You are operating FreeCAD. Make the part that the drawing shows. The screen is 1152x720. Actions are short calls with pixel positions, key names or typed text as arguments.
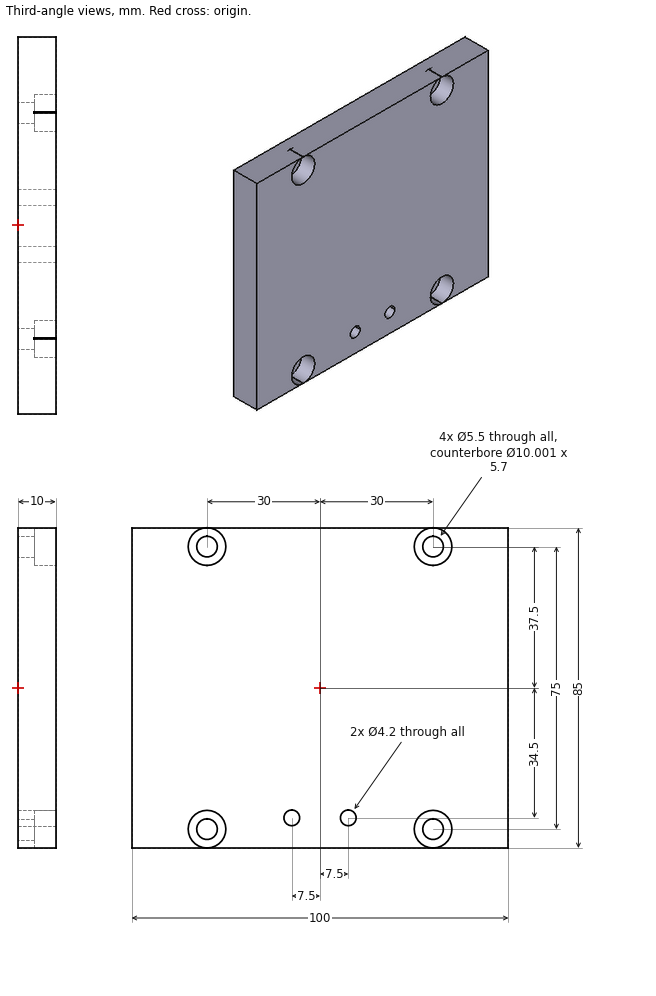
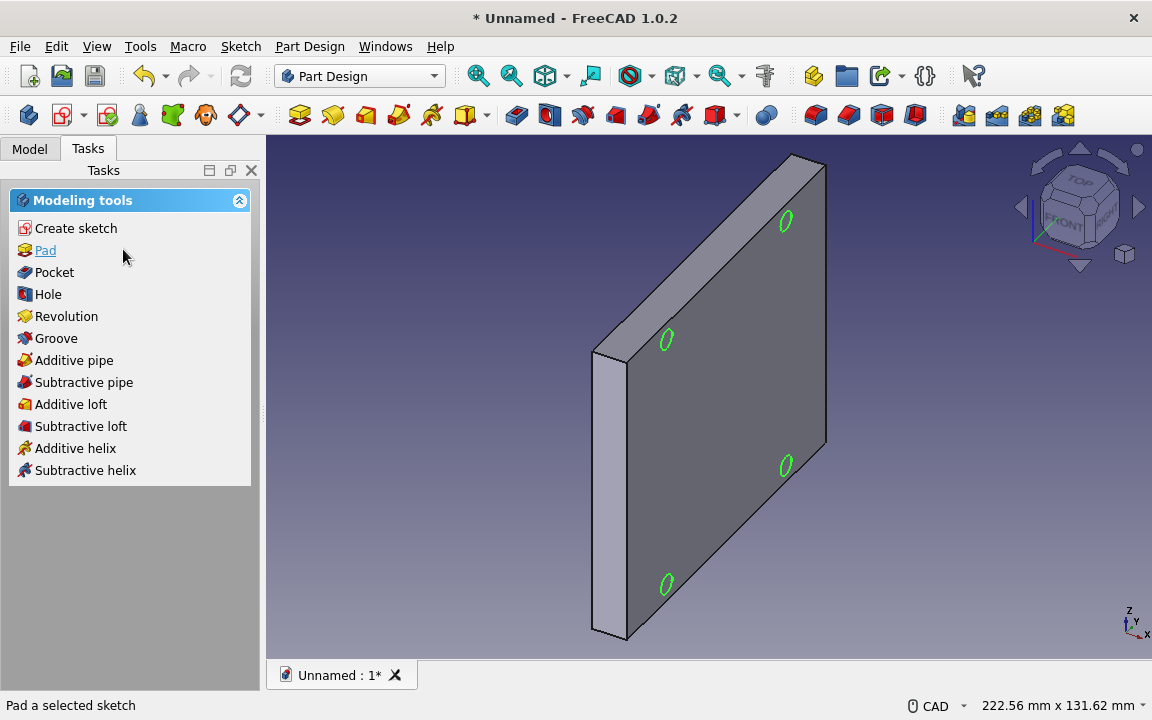
click(550, 116)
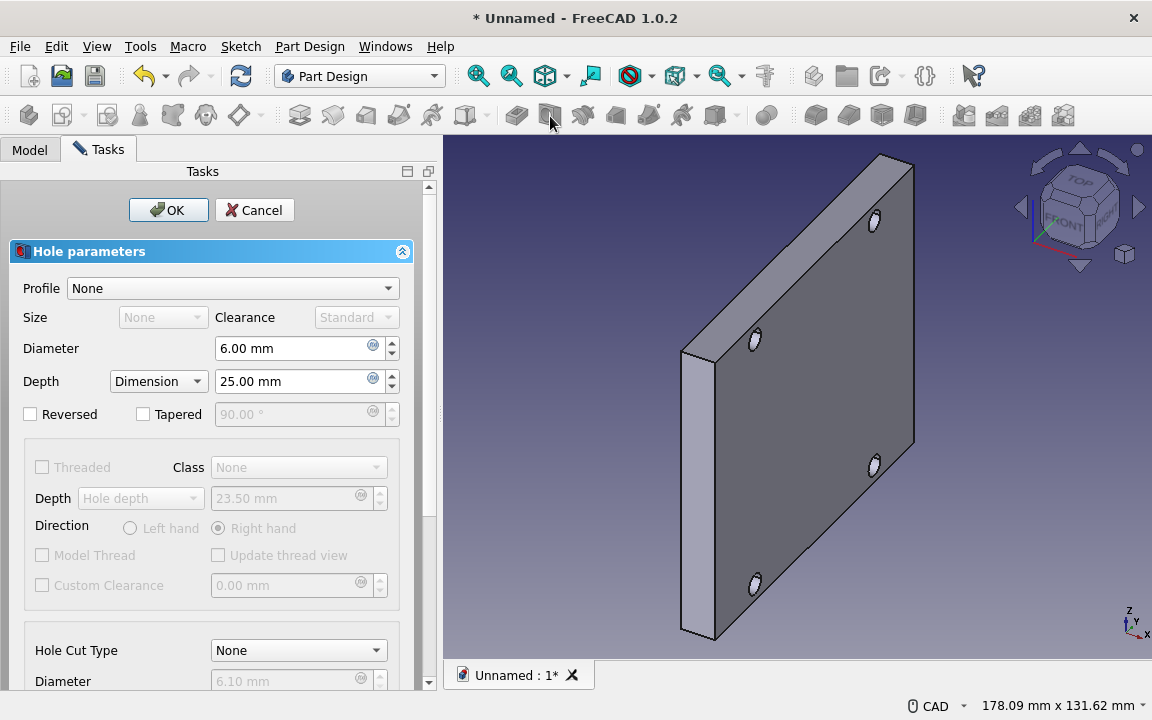
triple_click(300, 348)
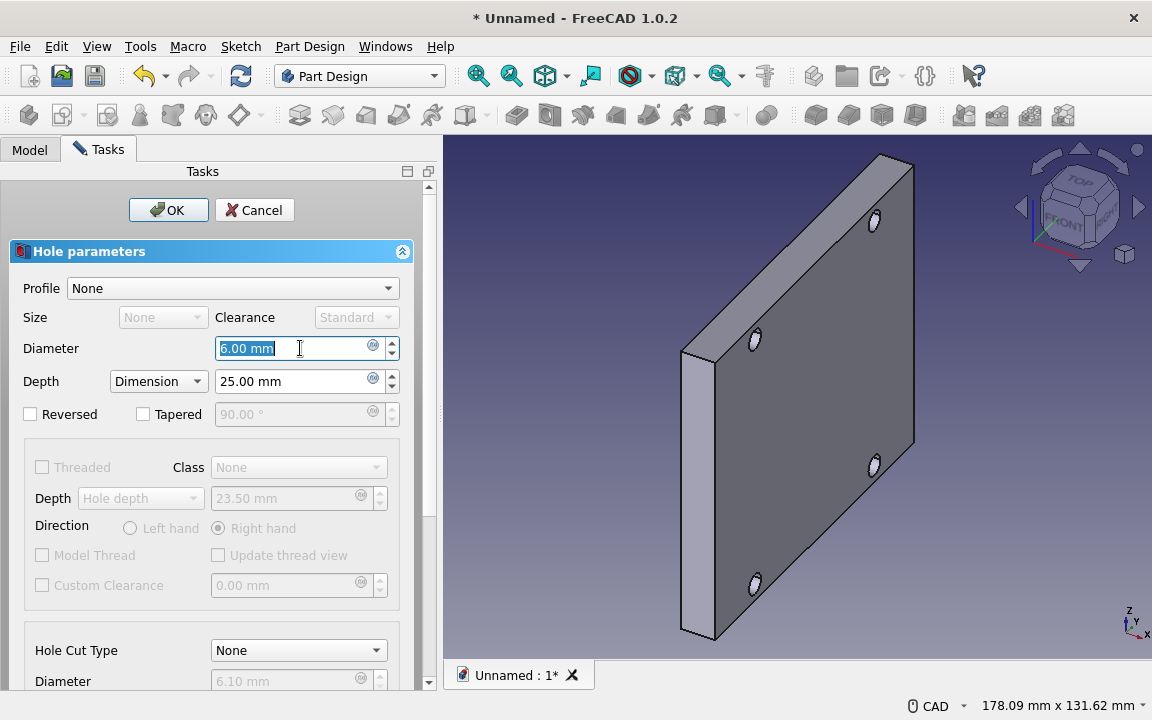
text(5.5)
key(Tab)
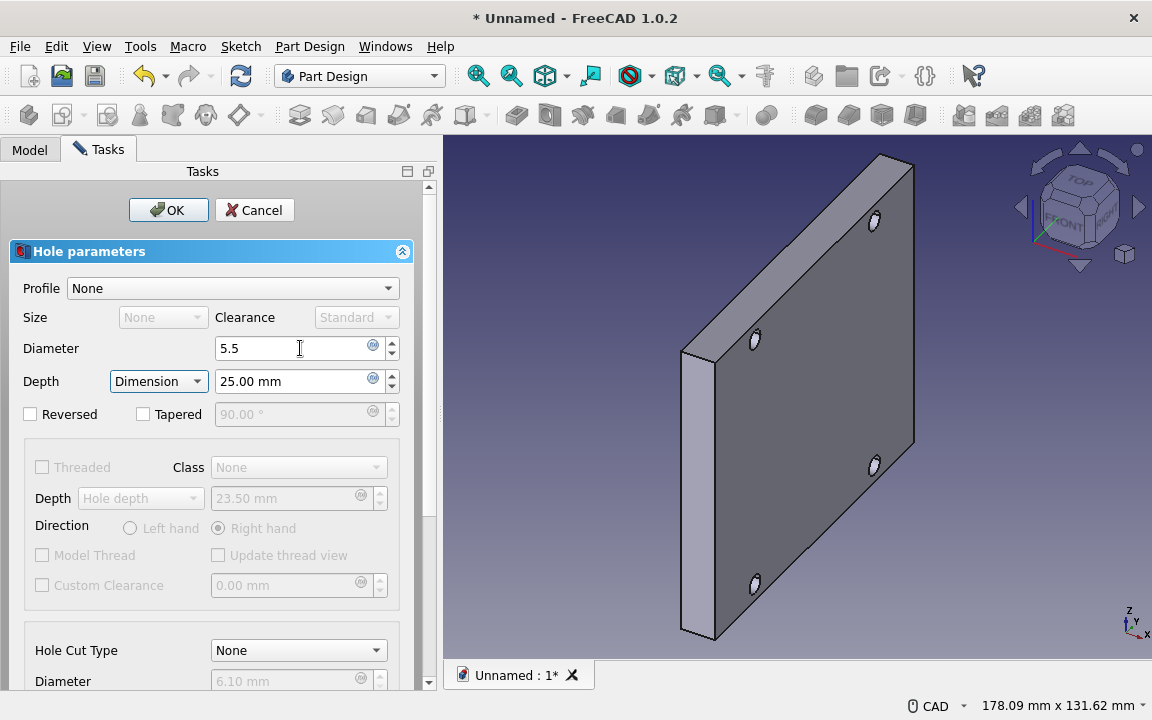
click(160, 382)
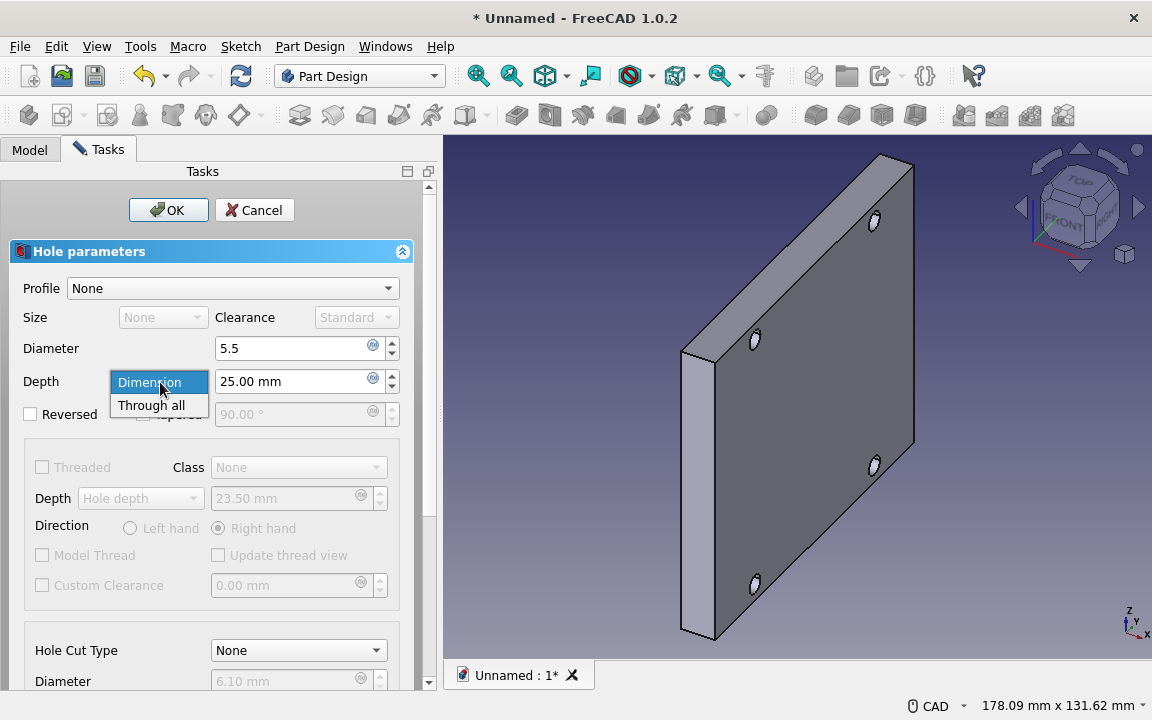
click(158, 406)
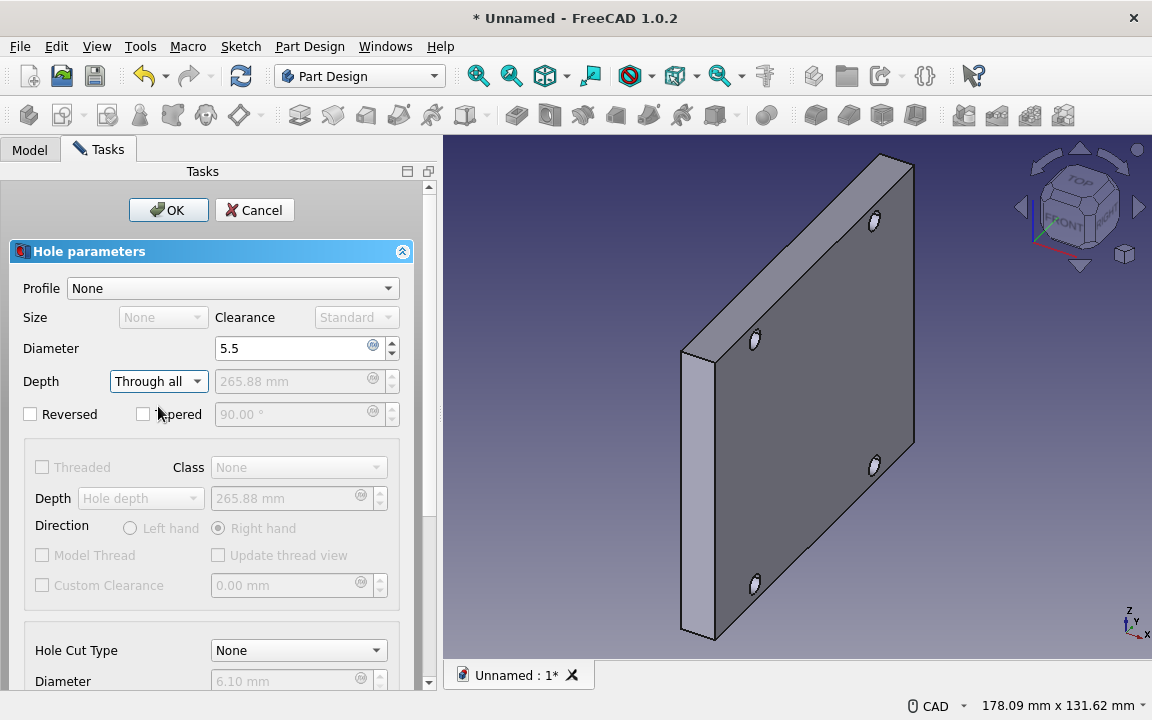
click(300, 650)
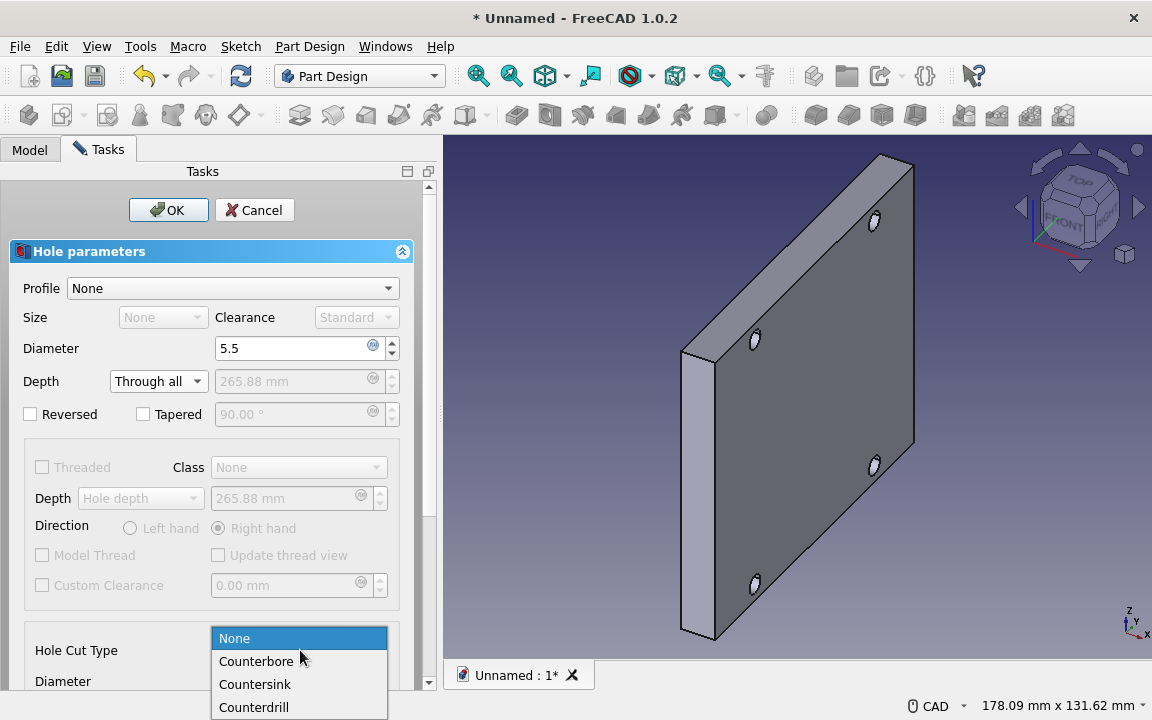
click(298, 662)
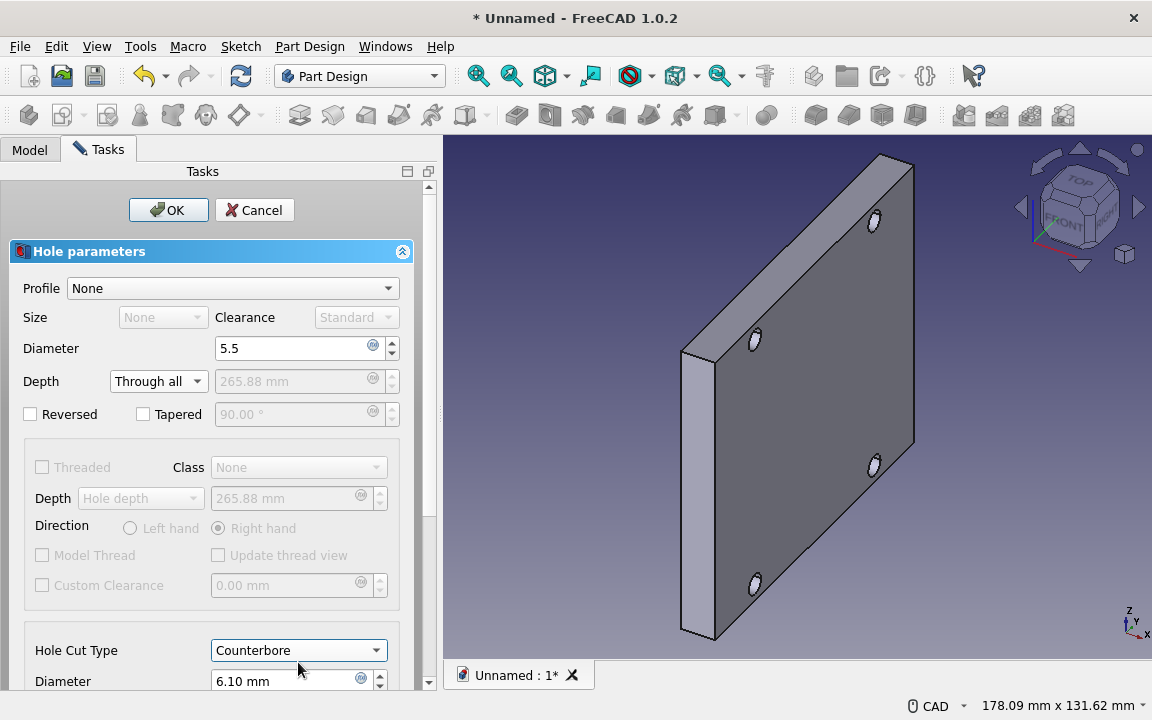
scroll(429, 436, down, 2)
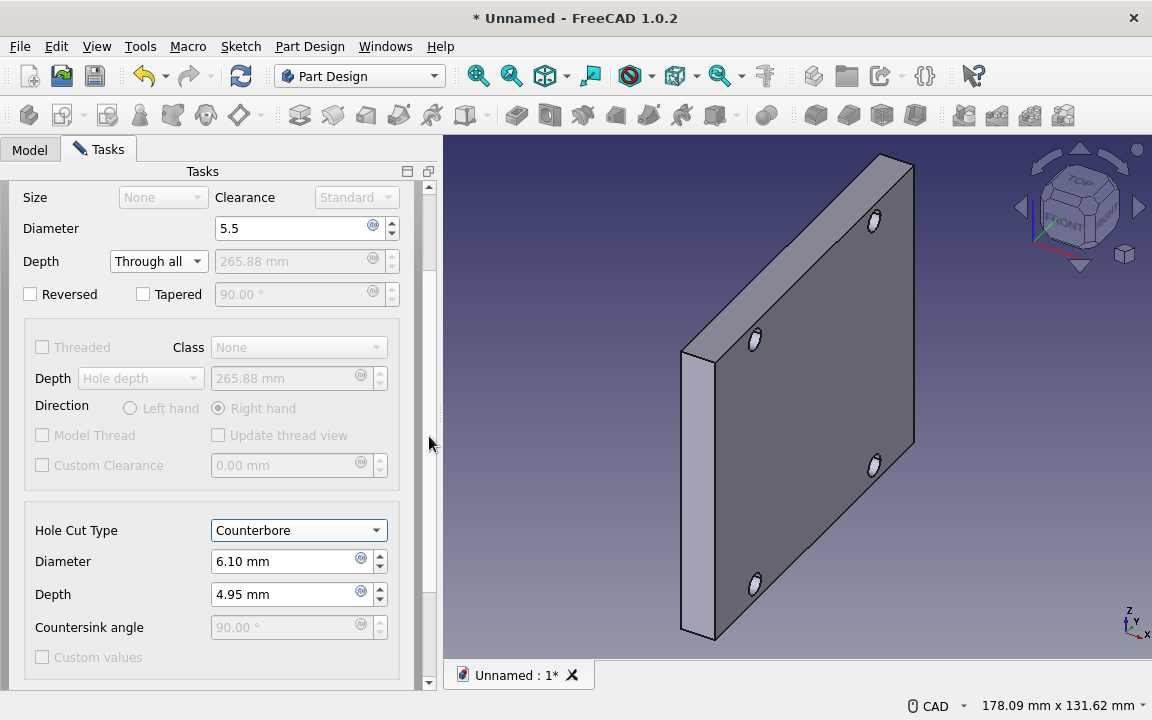
triple_click(292, 562)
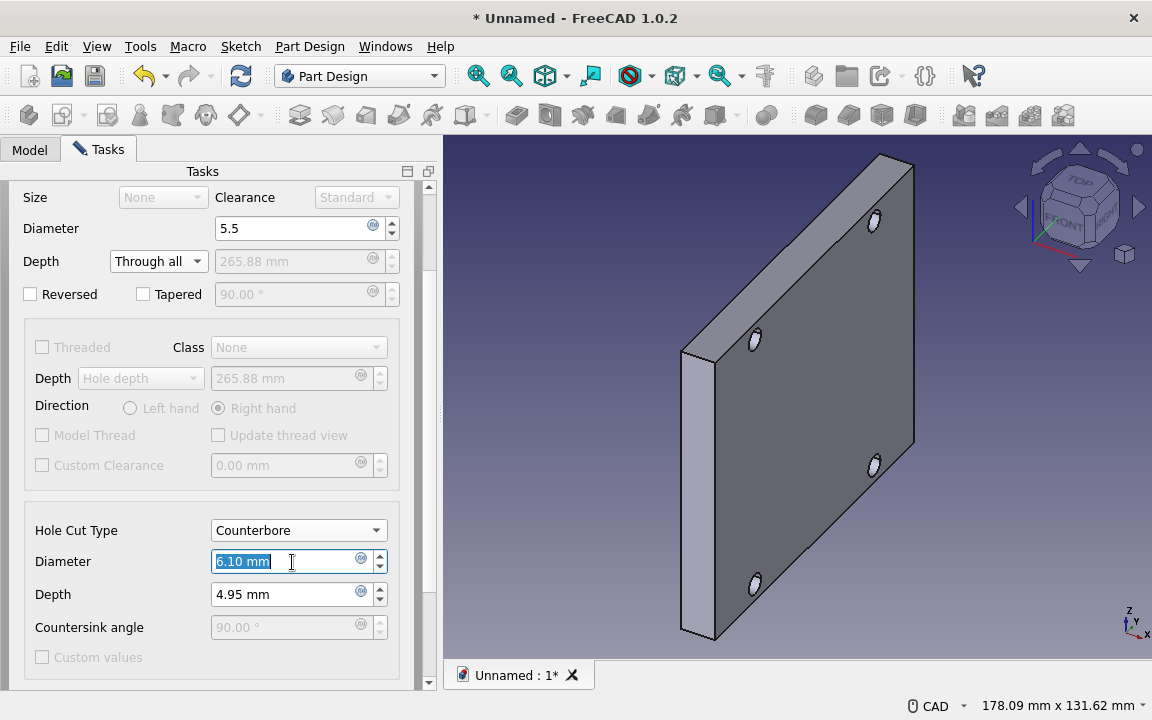
text(10.001)
key(Tab)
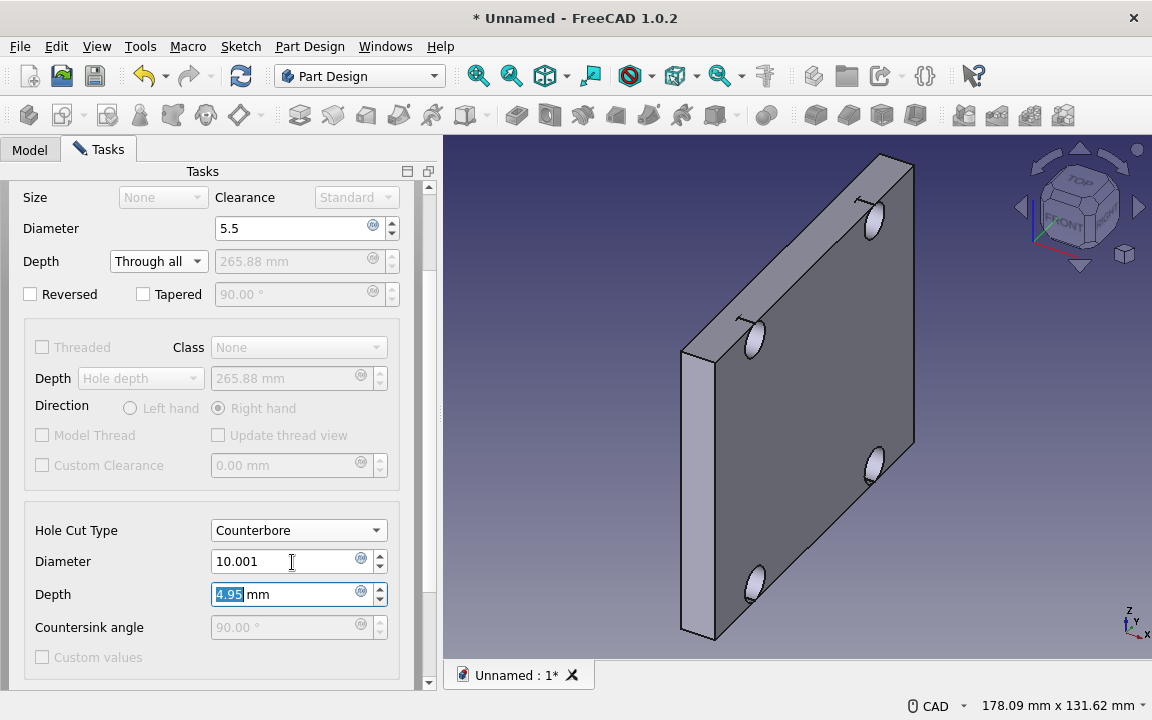
text(5.7)
key(Tab)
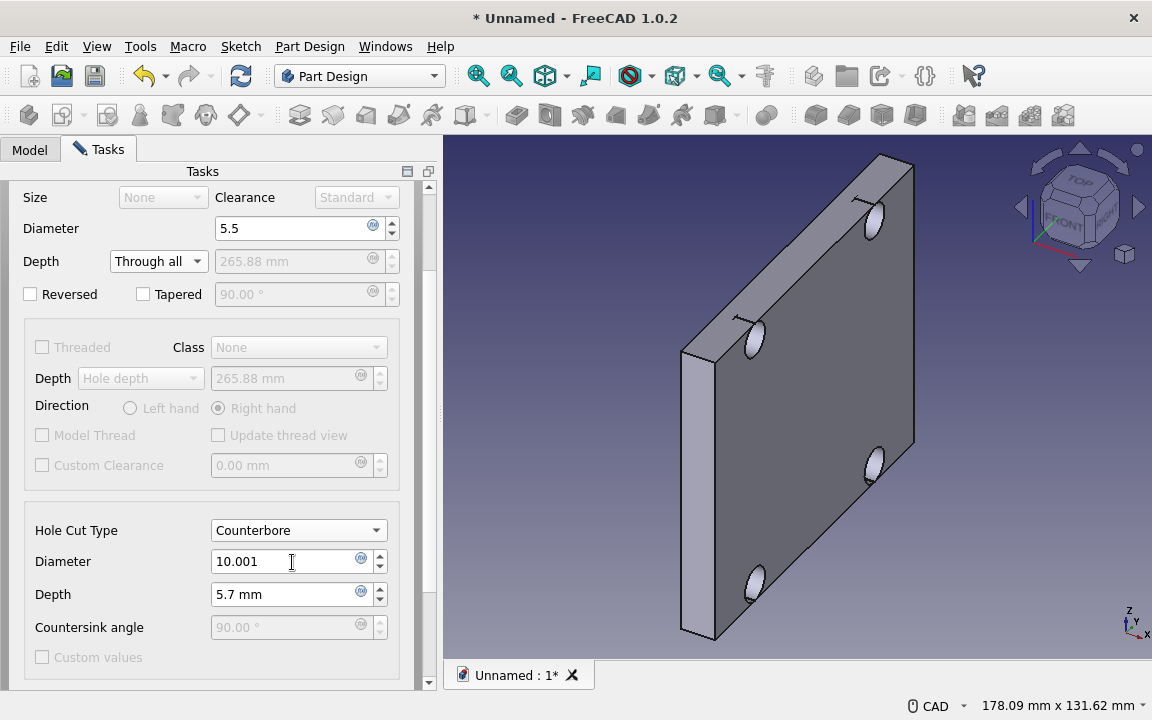
scroll(429, 436, up, 3)